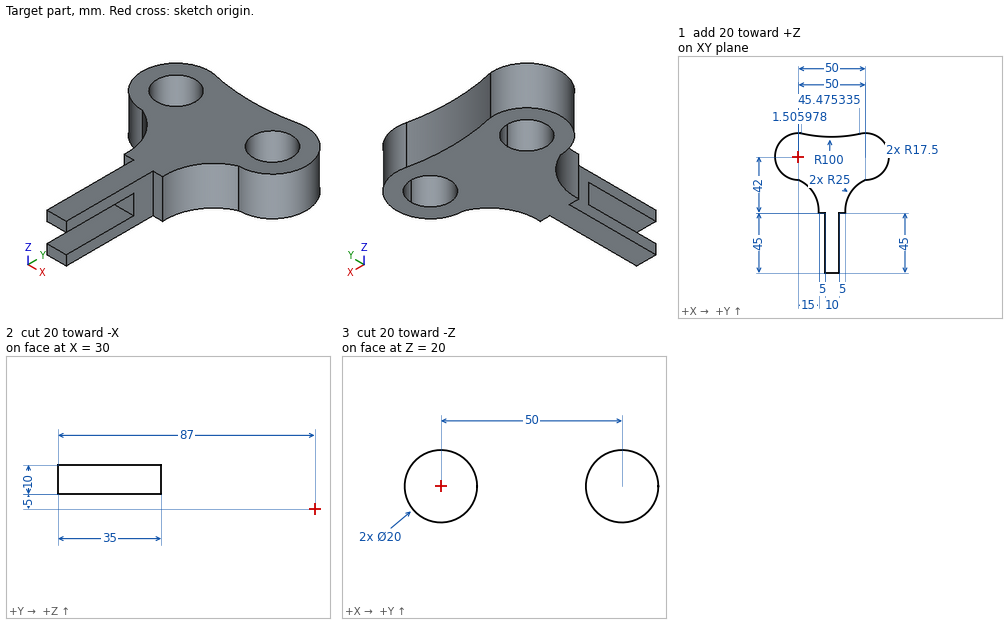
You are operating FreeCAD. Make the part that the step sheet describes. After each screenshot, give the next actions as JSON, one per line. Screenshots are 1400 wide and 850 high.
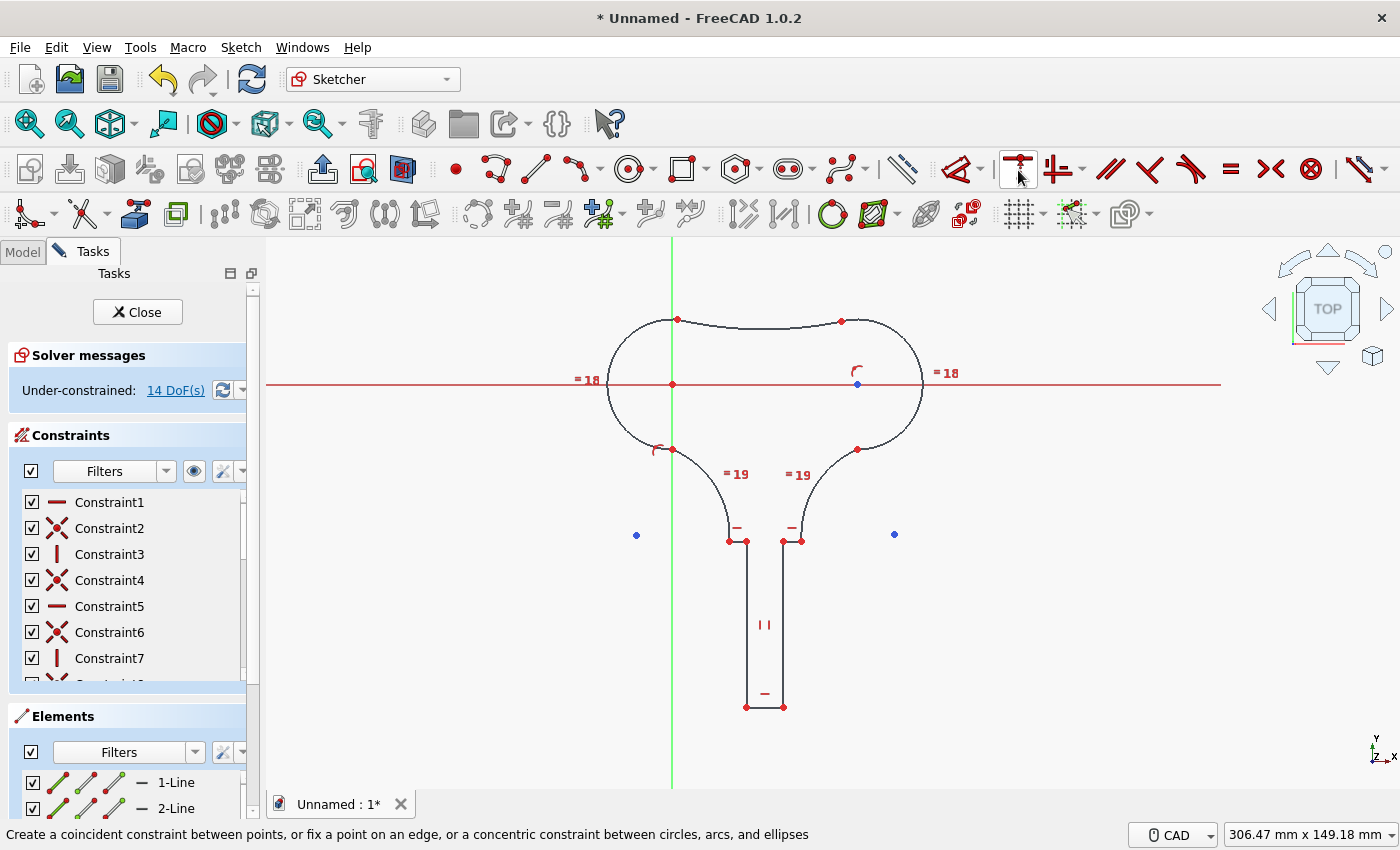
{"action": "left_click", "coordinate": [956, 170]}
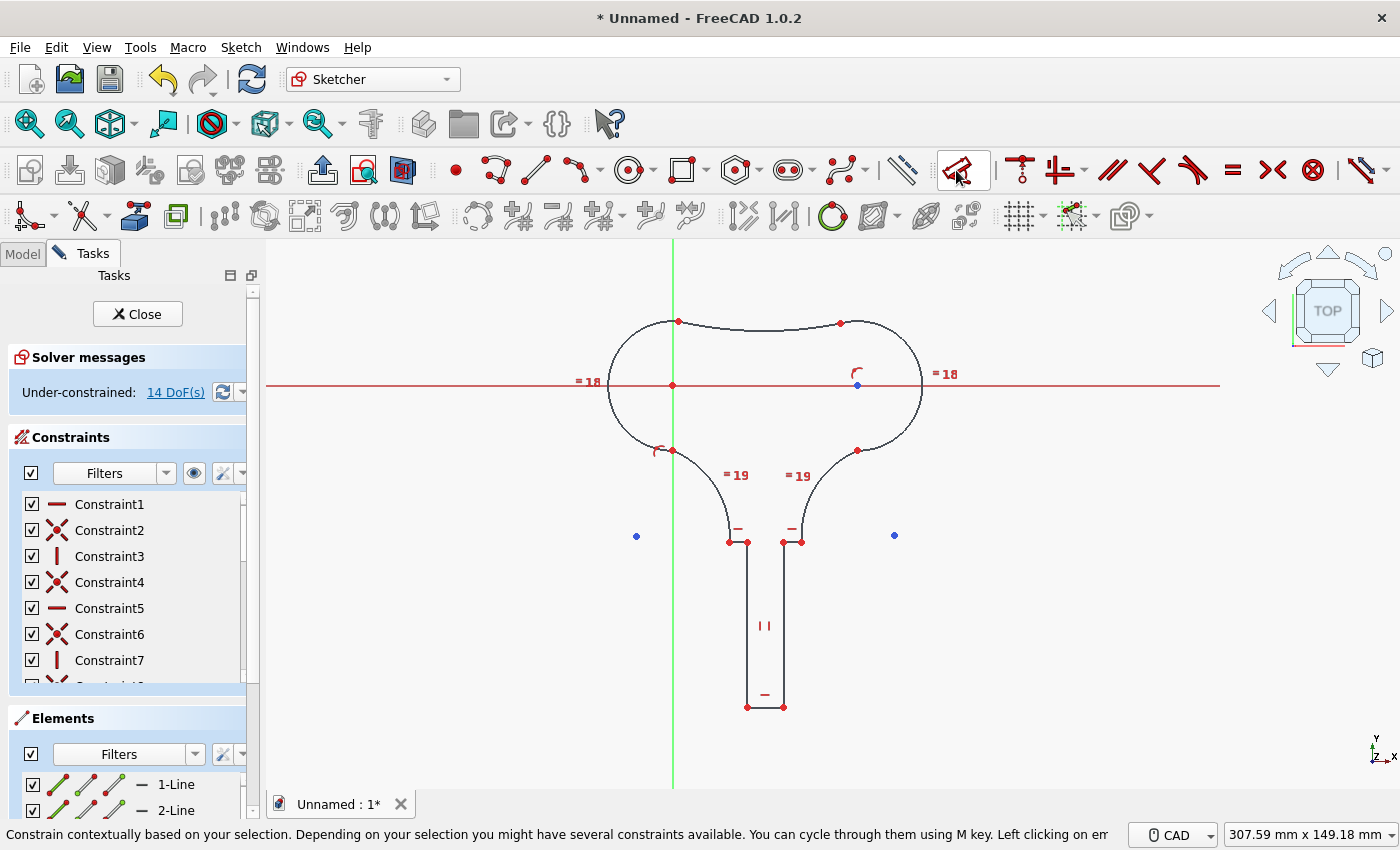
{"action": "left_click", "coordinate": [829, 470]}
{"action": "left_click", "coordinate": [806, 447]}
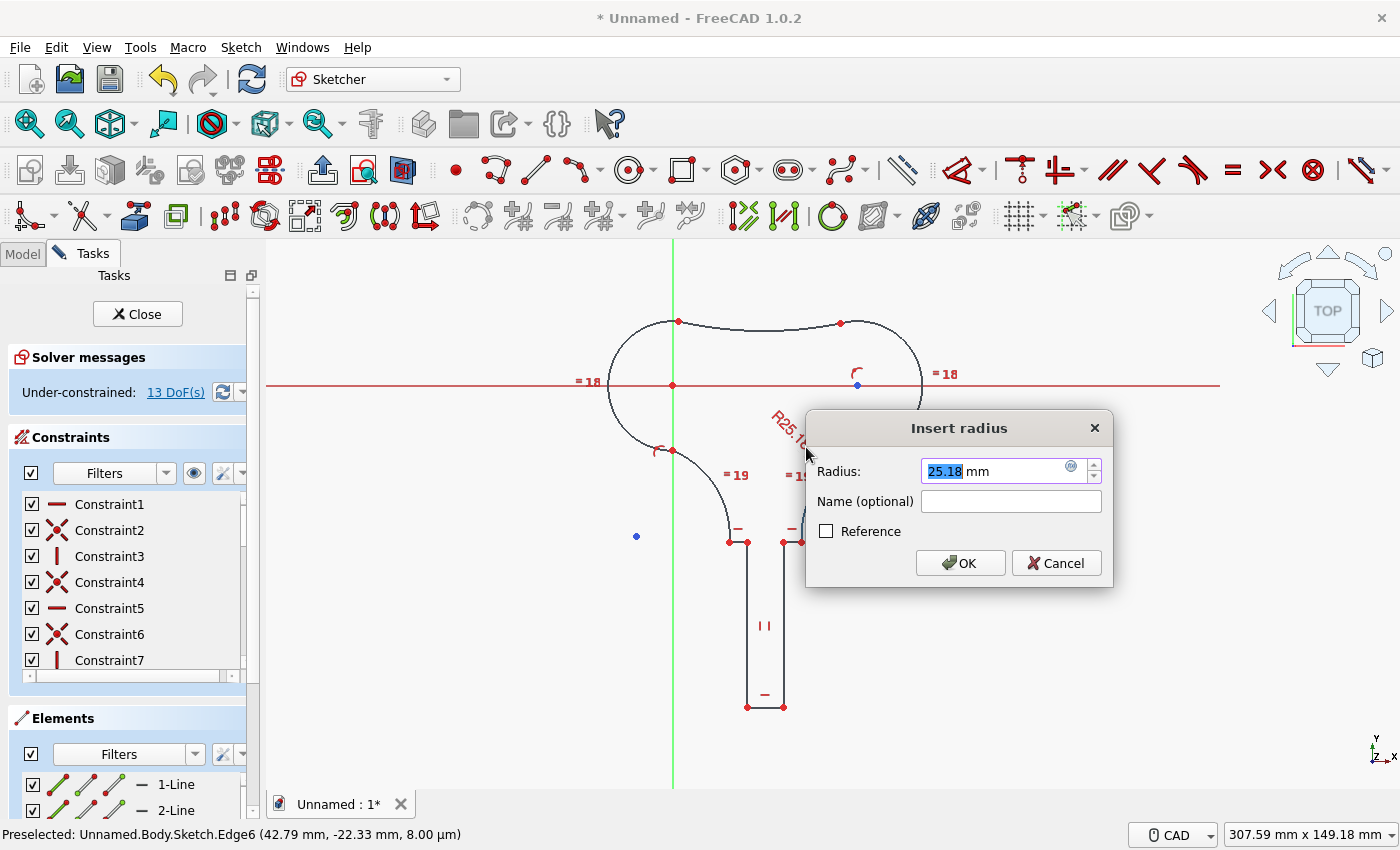
{"action": "type", "text": "25"}
{"action": "key", "text": "Return"}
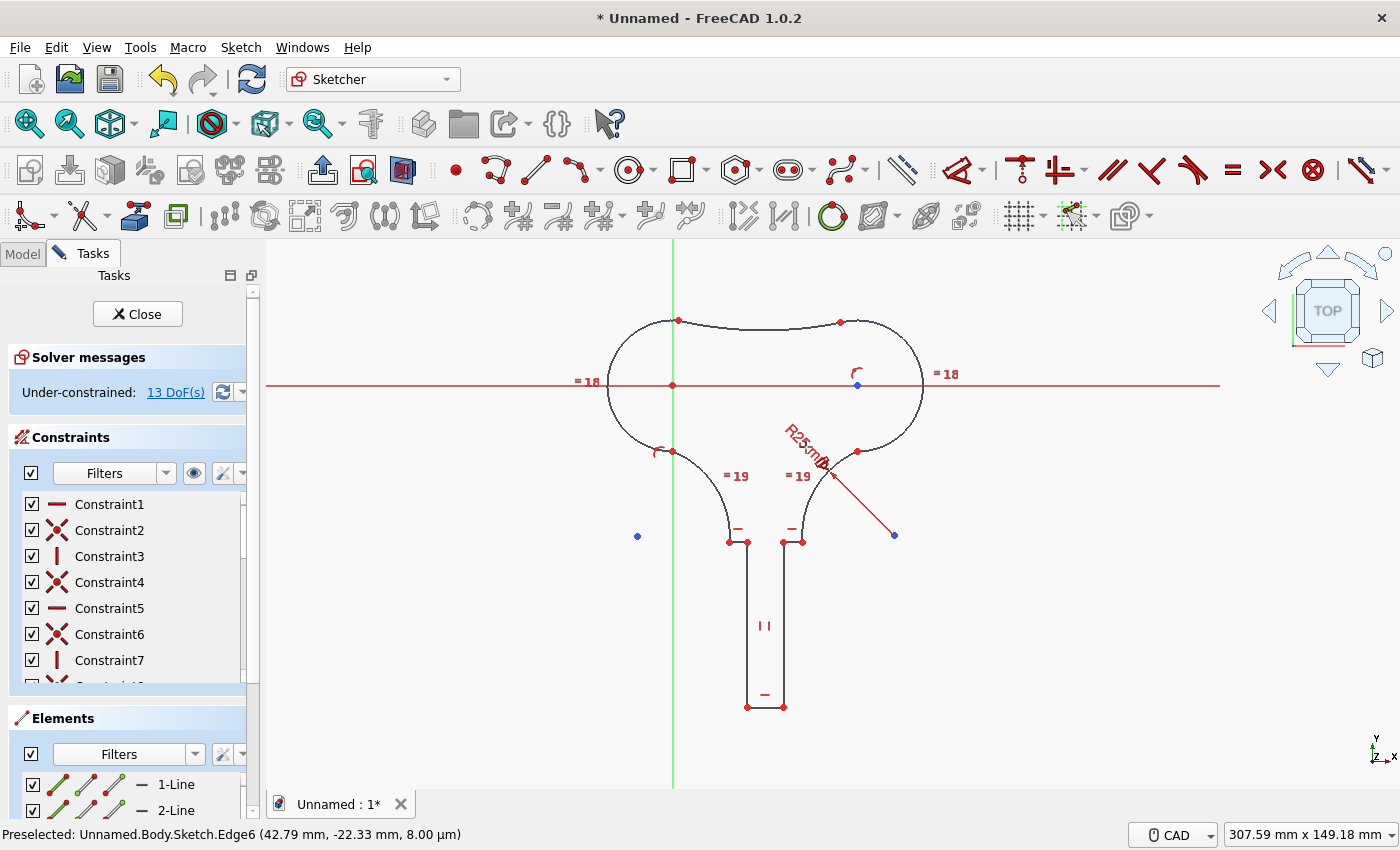
{"action": "left_click", "coordinate": [913, 420]}
{"action": "left_click", "coordinate": [940, 437]}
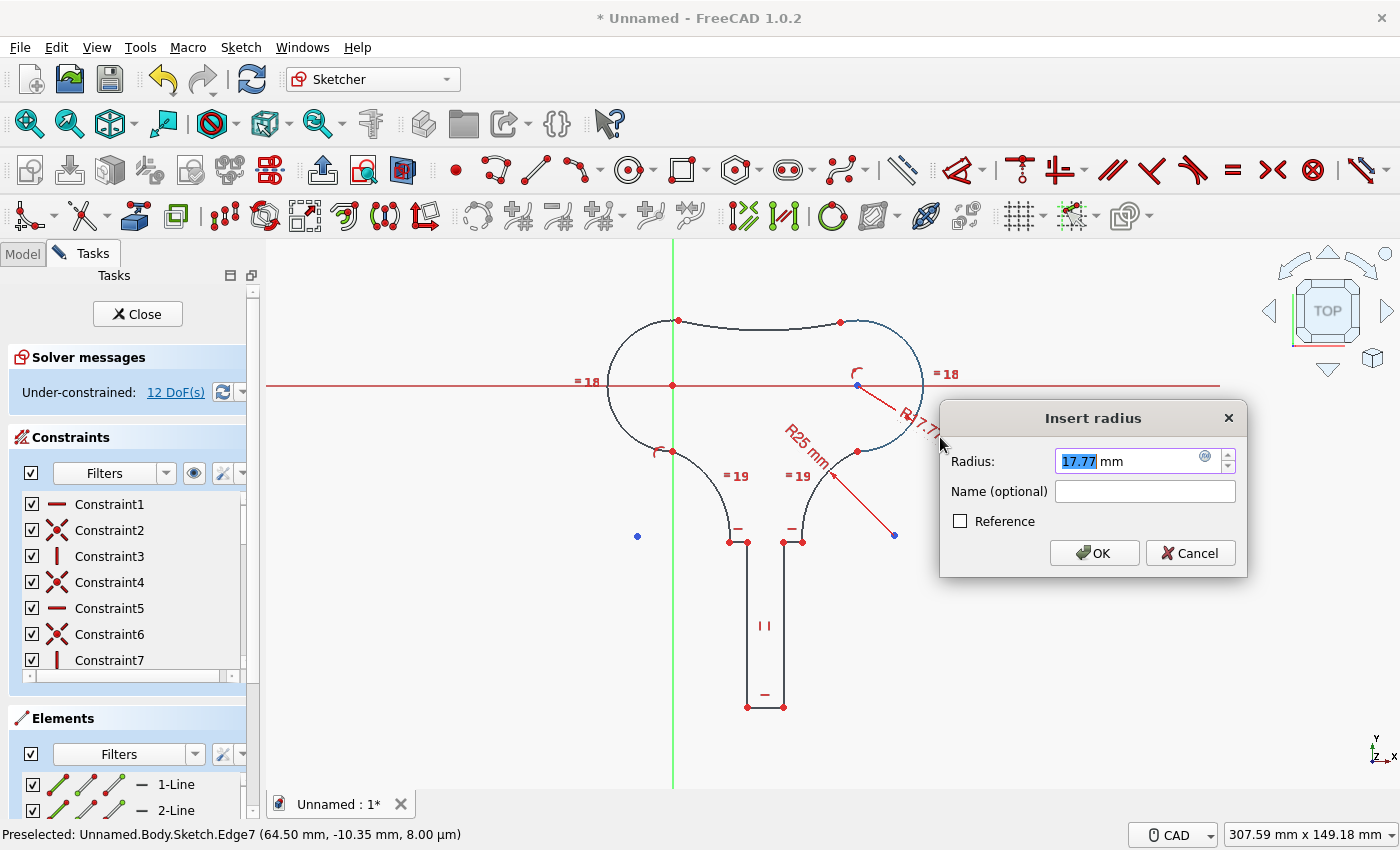
{"action": "type", "text": "17.5"}
{"action": "key", "text": "Return"}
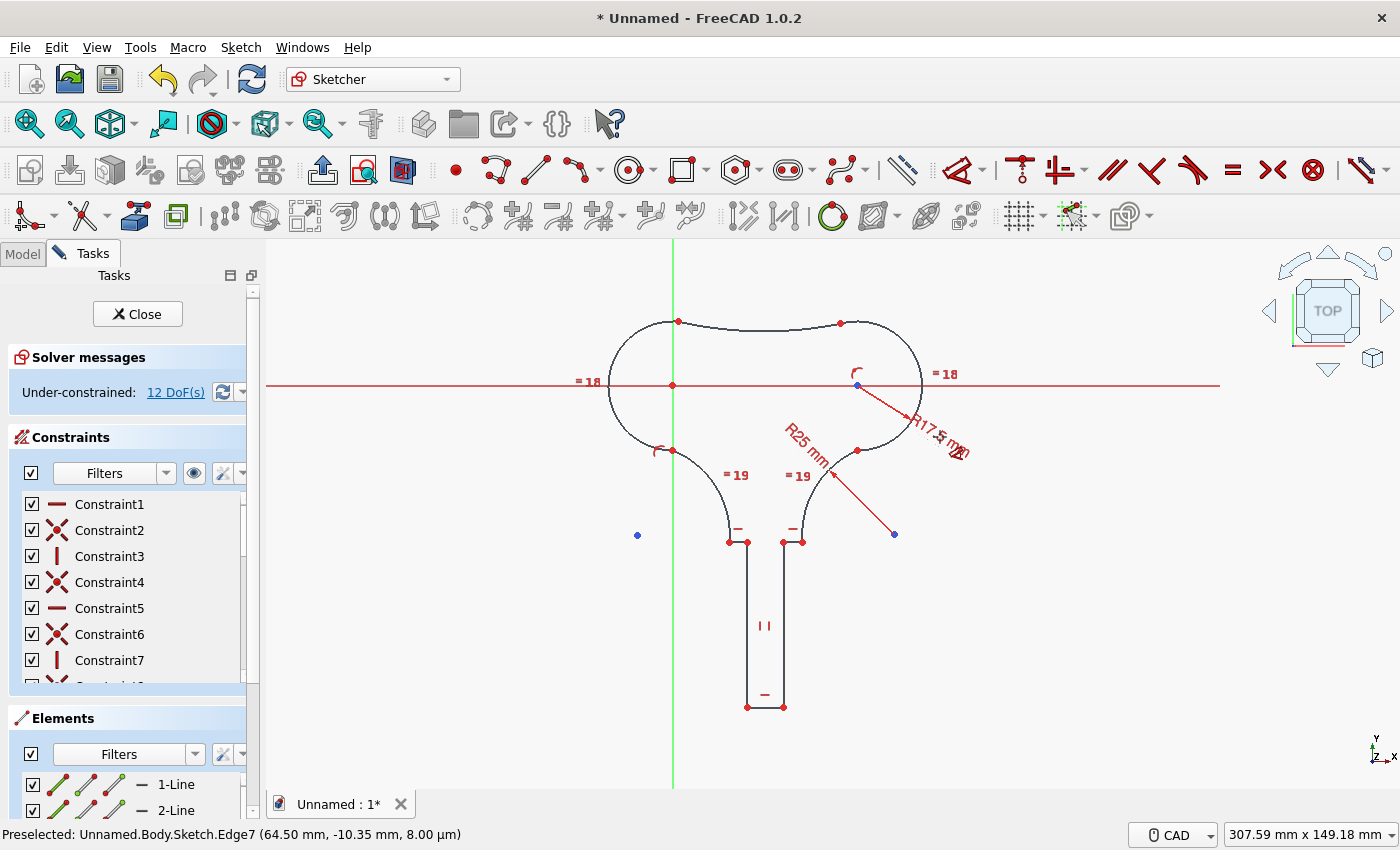
{"action": "left_click", "coordinate": [727, 330]}
{"action": "left_click", "coordinate": [724, 362]}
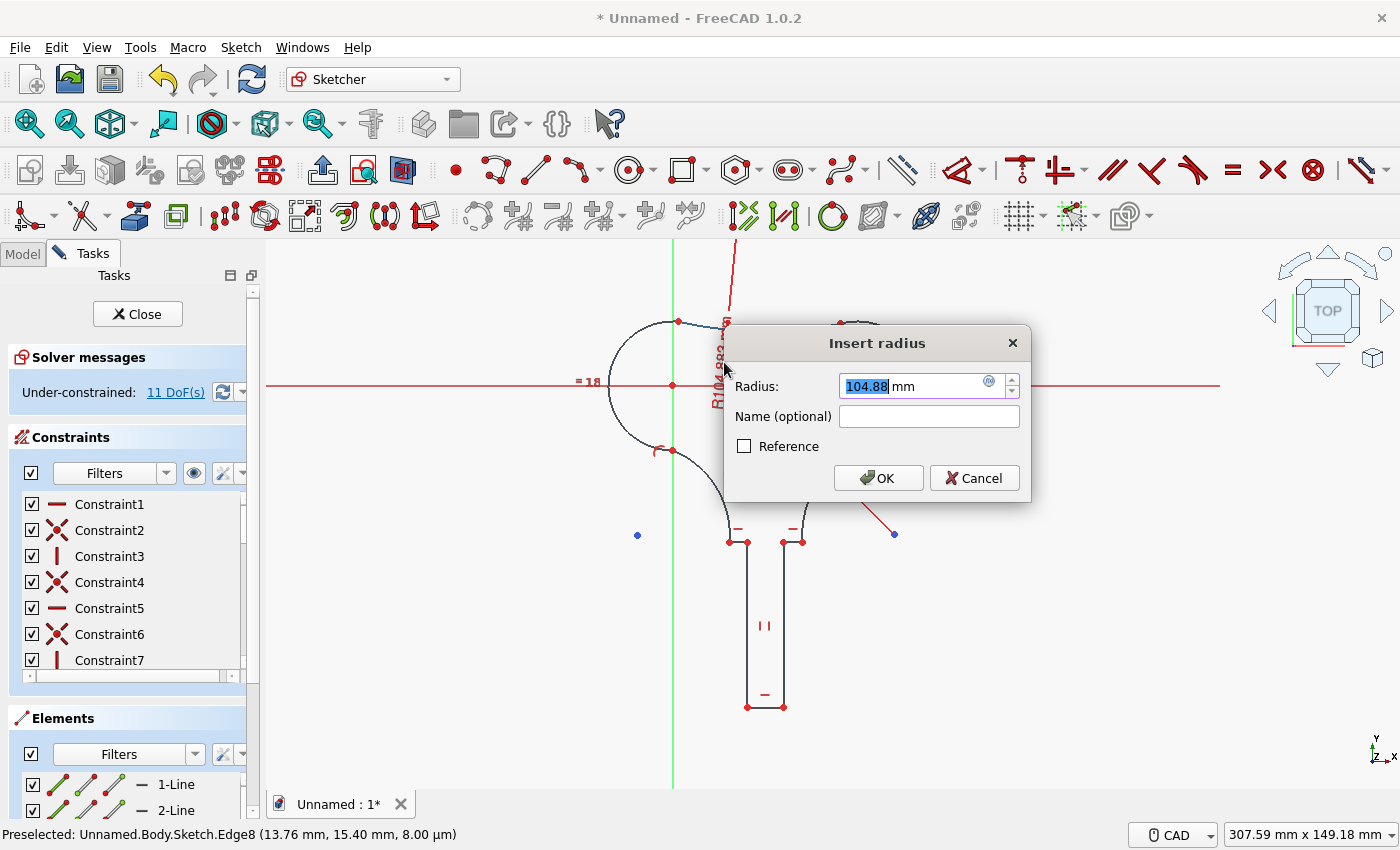
{"action": "type", "text": "100"}
{"action": "key", "text": "Return"}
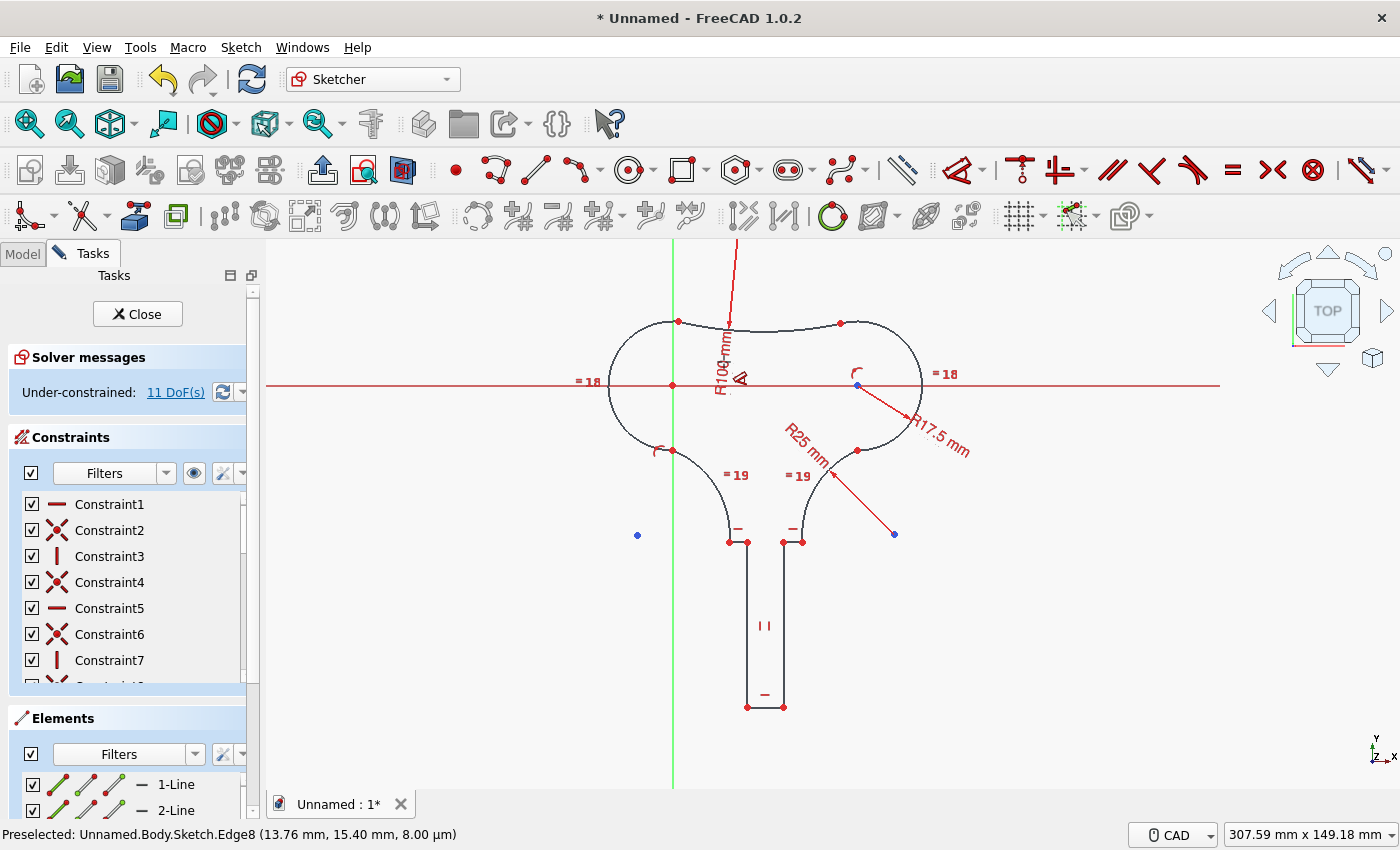
{"action": "scroll", "coordinate": [738, 542], "scroll_direction": "up", "scroll_amount": 4}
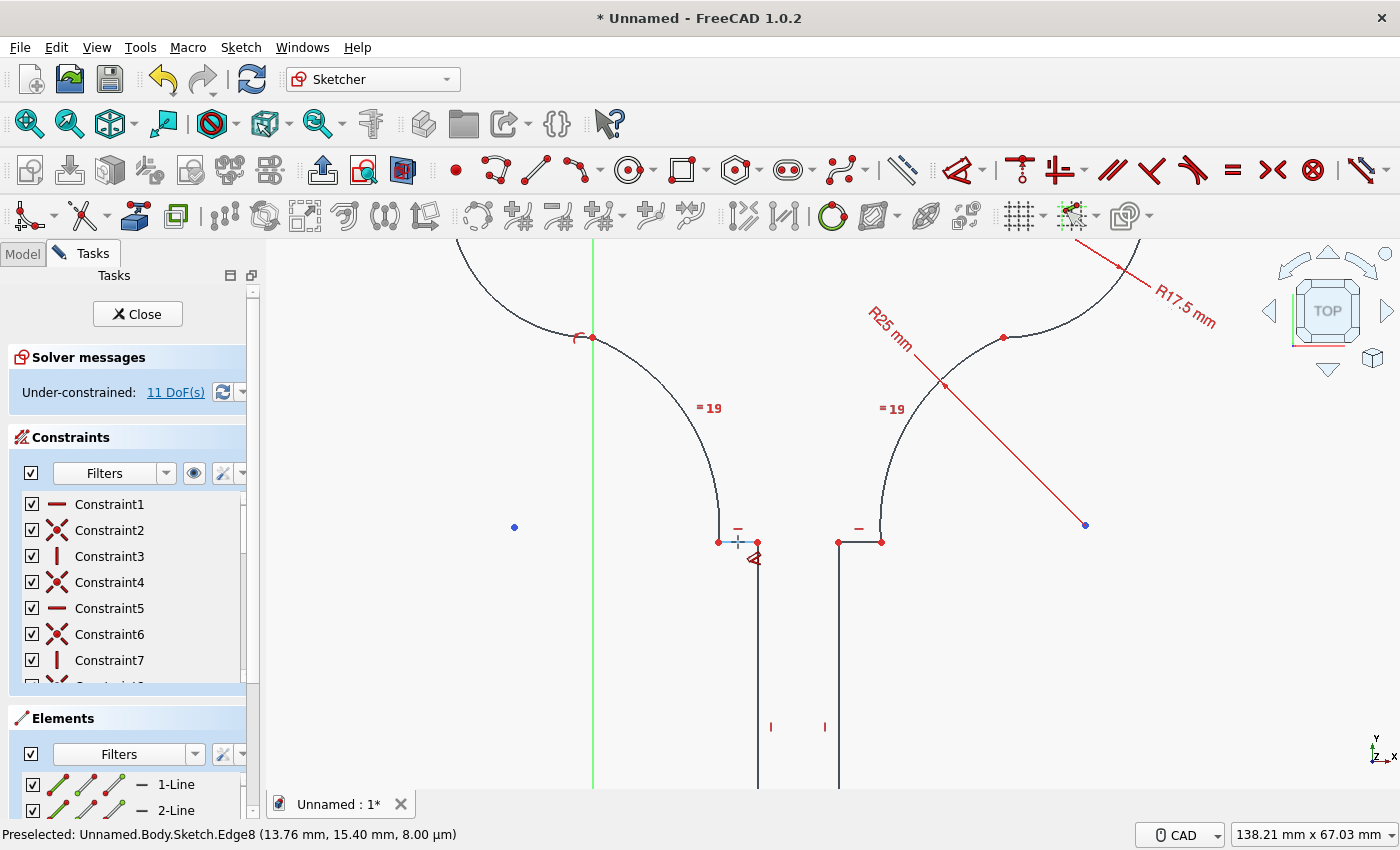
{"action": "left_click", "coordinate": [738, 542]}
{"action": "left_click", "coordinate": [738, 576]}